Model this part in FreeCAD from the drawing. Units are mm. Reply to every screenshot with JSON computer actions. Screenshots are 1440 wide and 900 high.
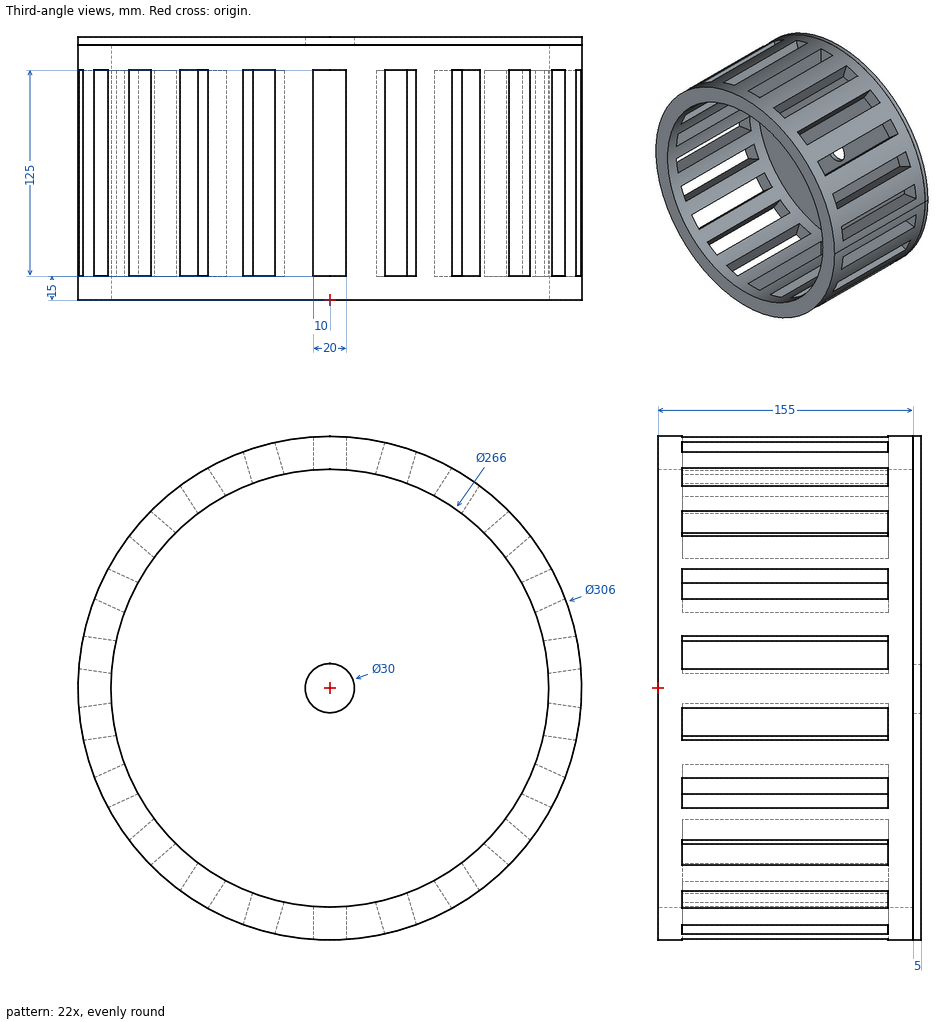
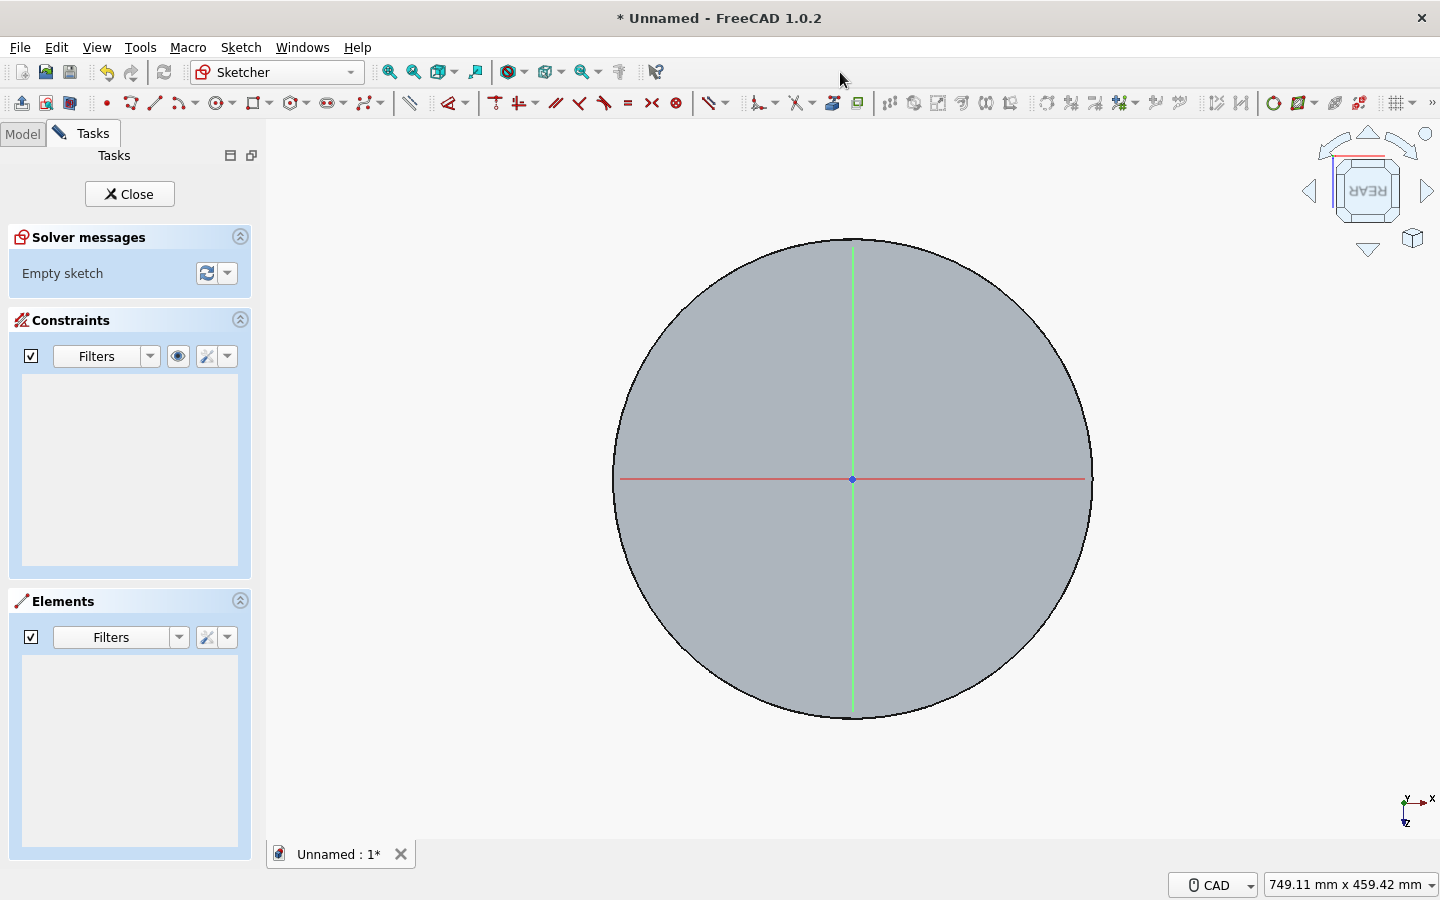
{"action": "scroll", "coordinate": [861, 479], "scroll_direction": "up", "scroll_amount": 11}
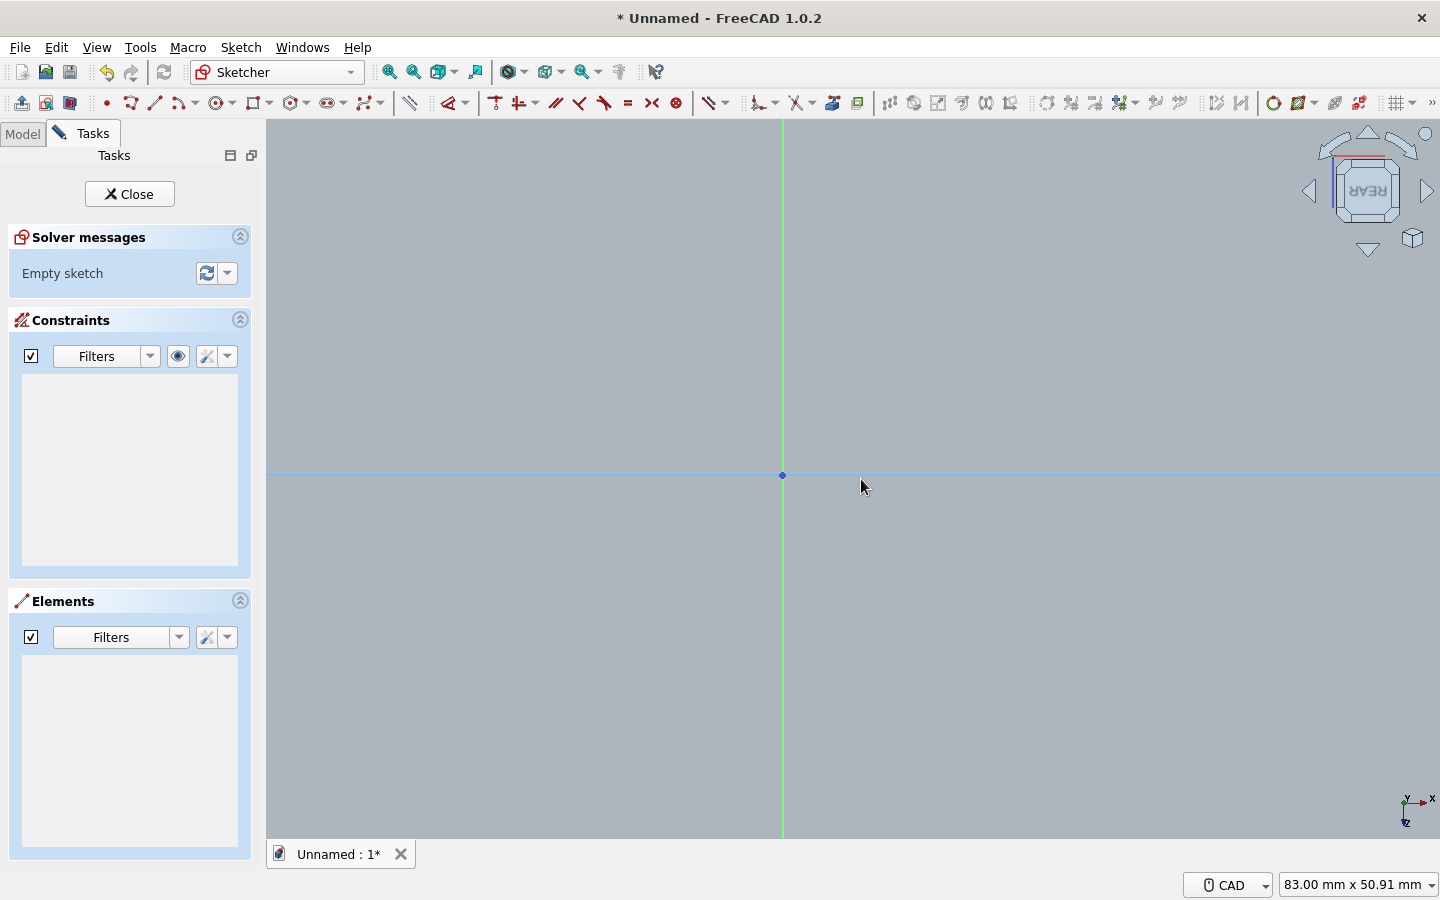
{"action": "left_click", "coordinate": [216, 104]}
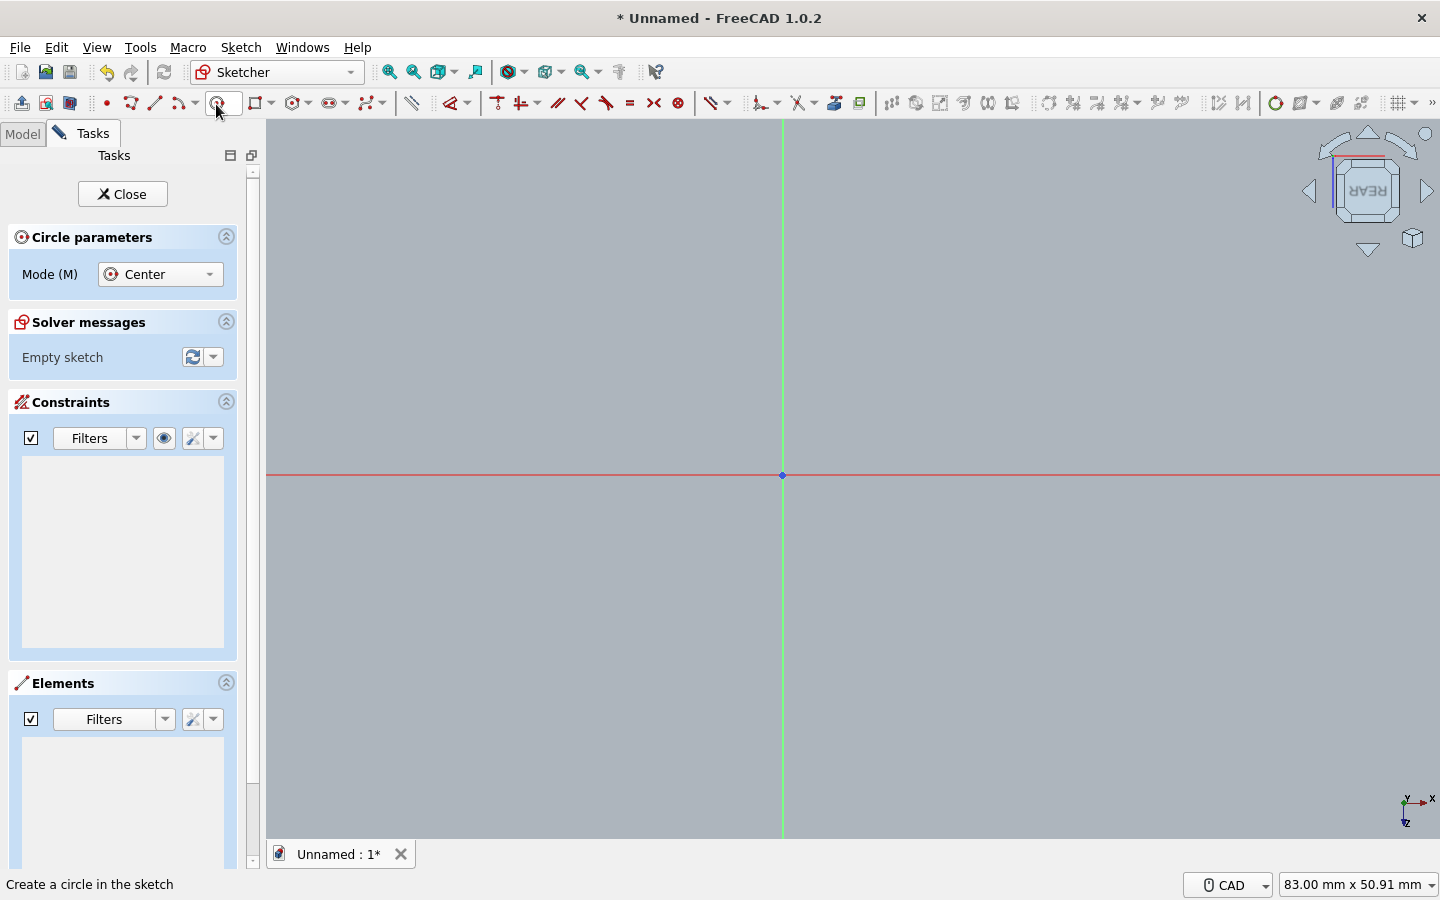
{"action": "left_click", "coordinate": [783, 475]}
{"action": "left_click", "coordinate": [933, 325]}
{"action": "key", "text": "Escape"}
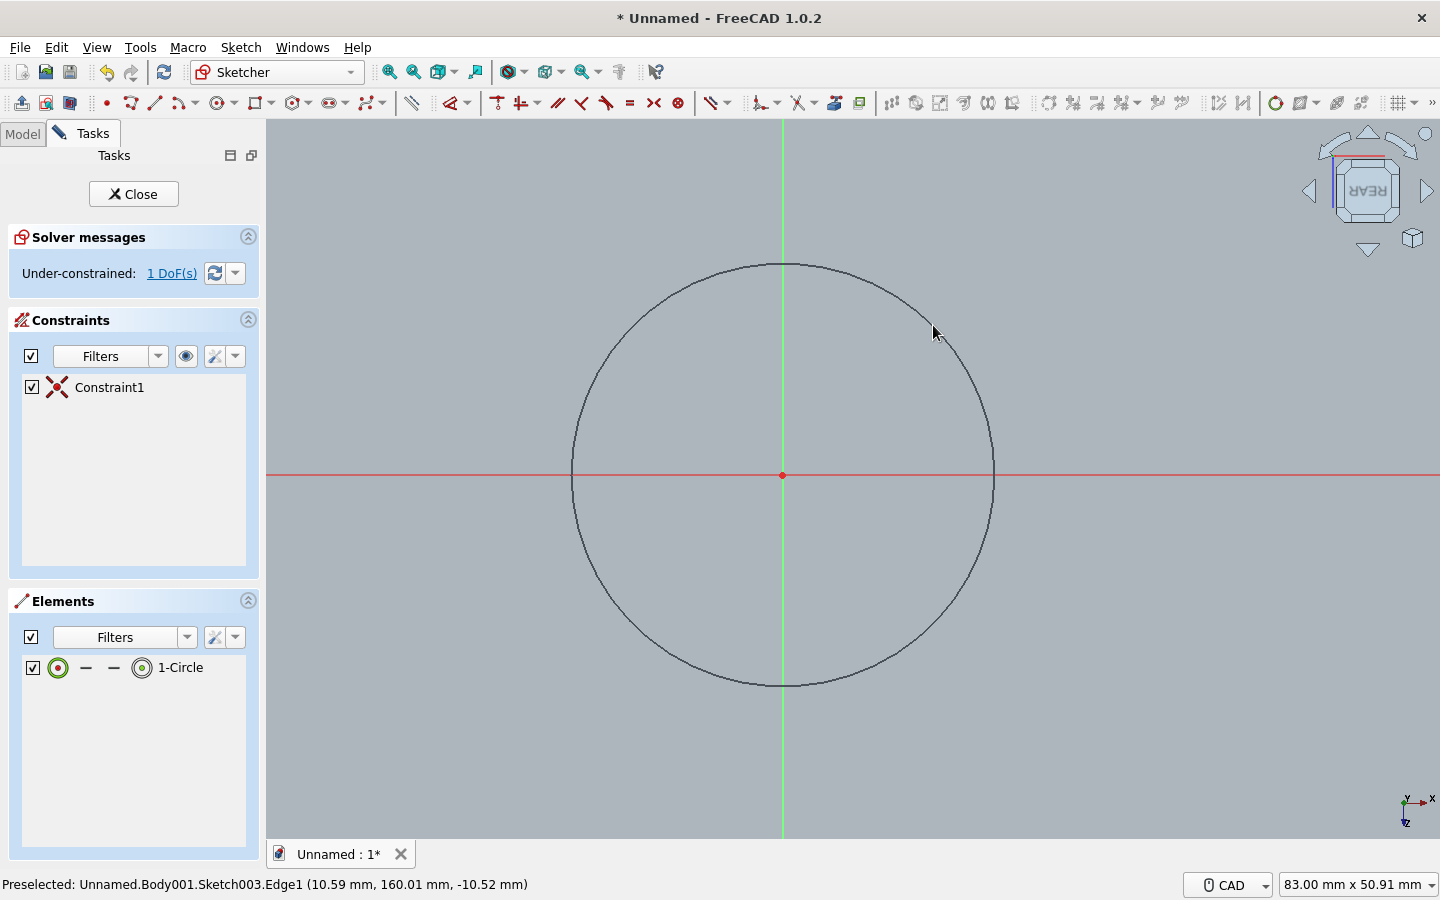
{"action": "left_click", "coordinate": [450, 104]}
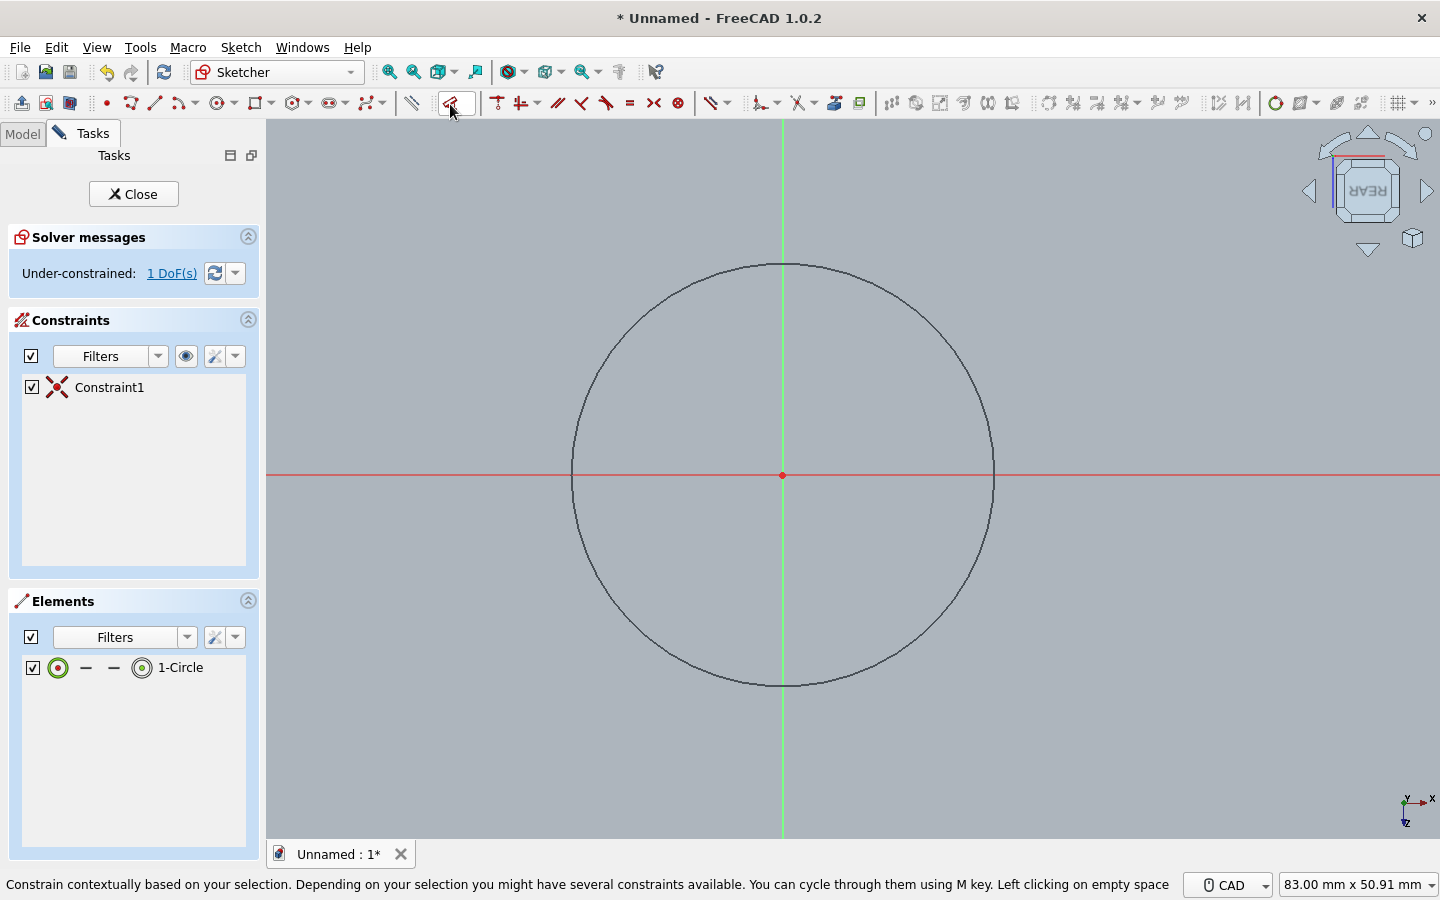
{"action": "left_click", "coordinate": [932, 325]}
{"action": "left_click", "coordinate": [955, 302]}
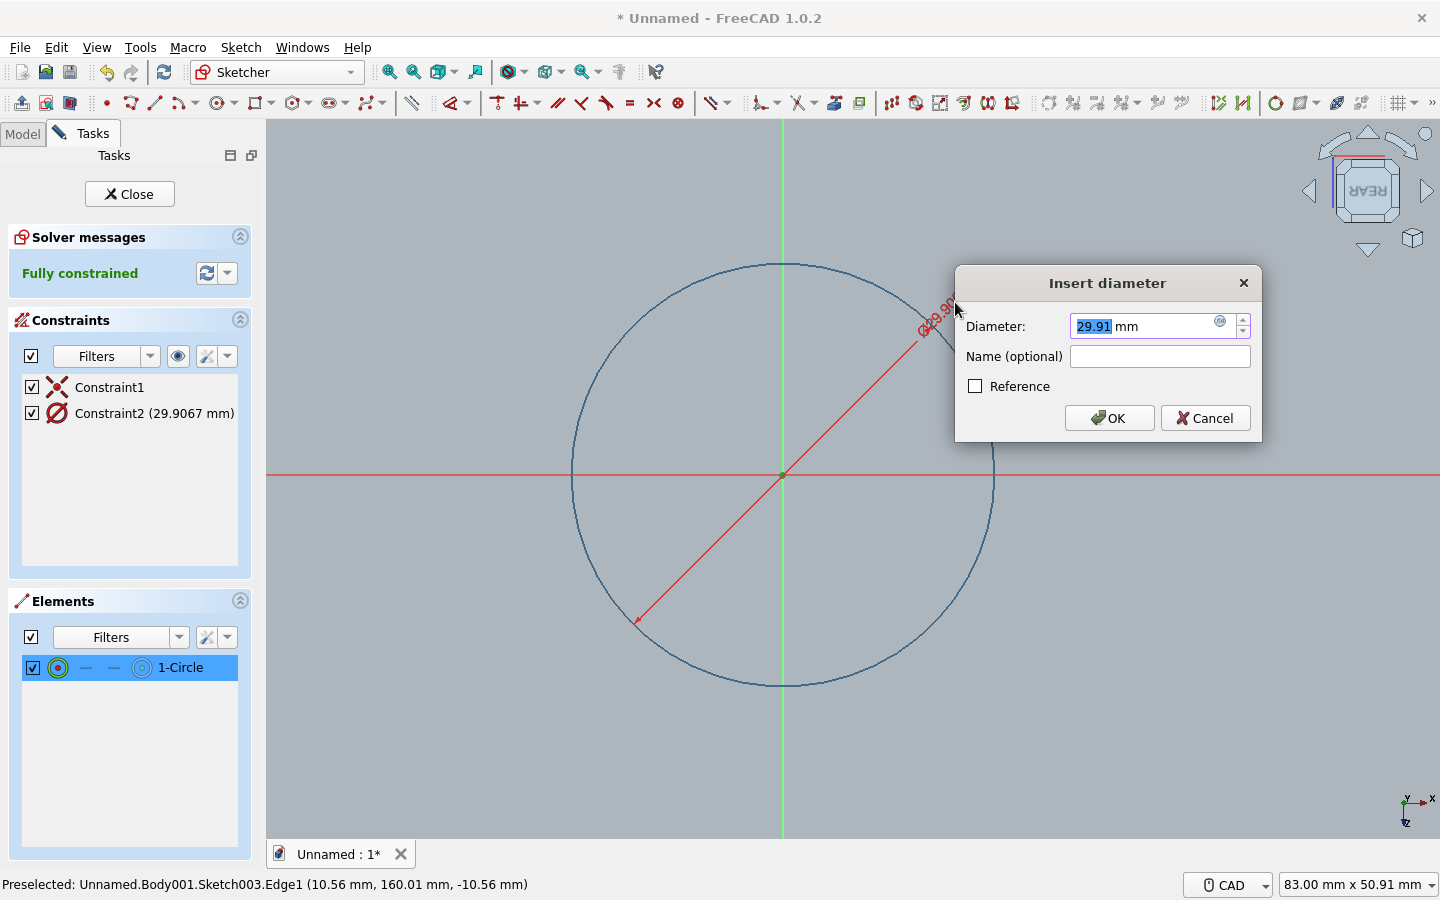
{"action": "type", "text": "30"}
{"action": "key", "text": "Return"}
{"action": "key", "text": "Escape"}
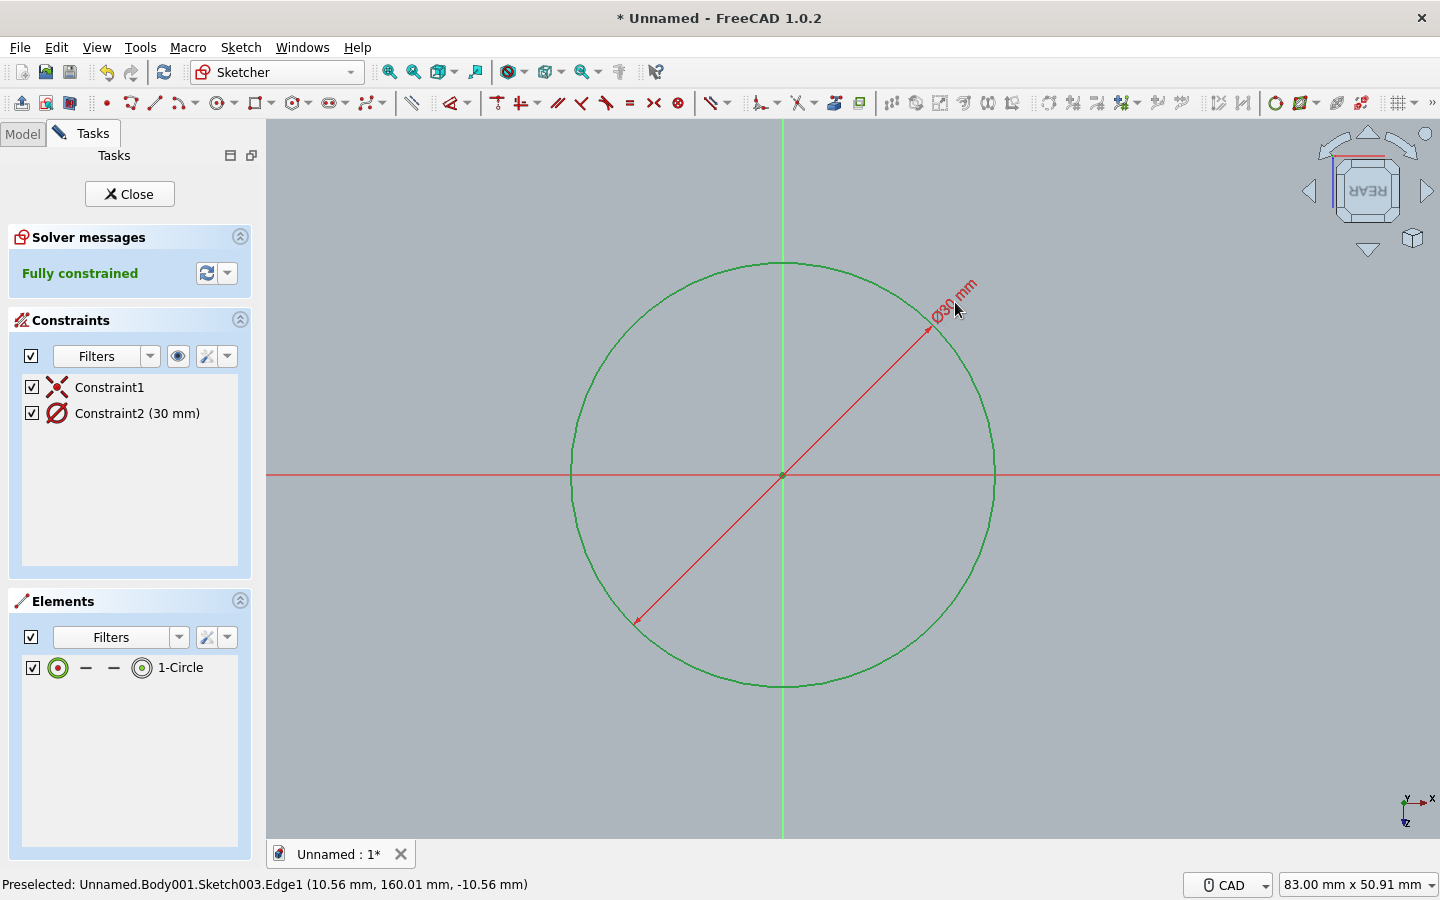
{"action": "left_click", "coordinate": [130, 194]}